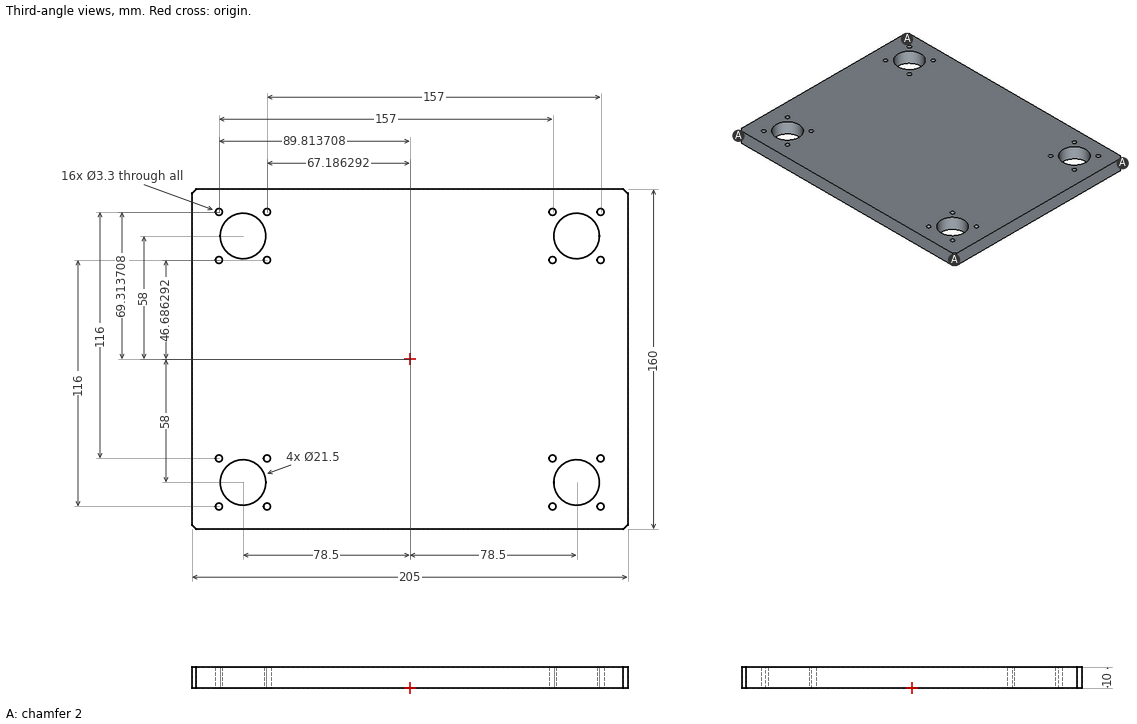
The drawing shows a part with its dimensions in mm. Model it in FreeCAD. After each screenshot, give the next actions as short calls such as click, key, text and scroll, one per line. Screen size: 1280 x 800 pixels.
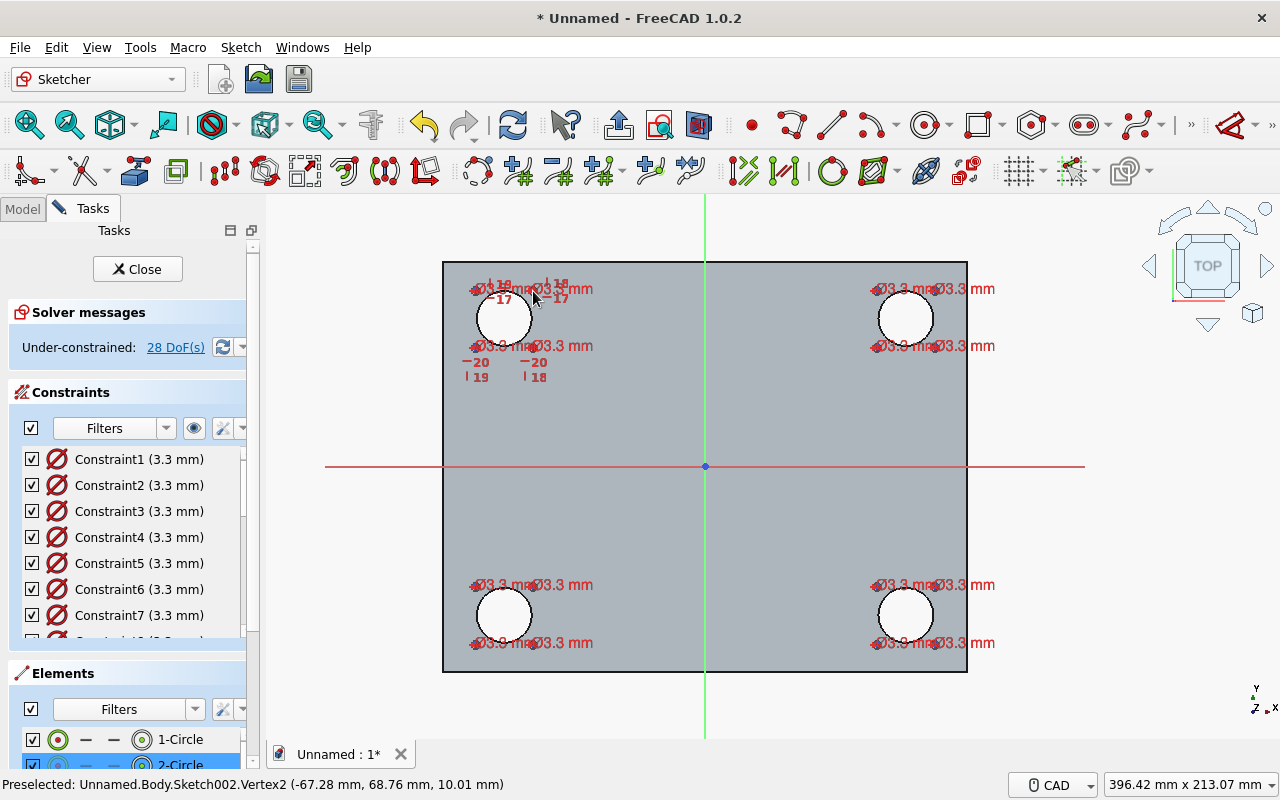
click(877, 291)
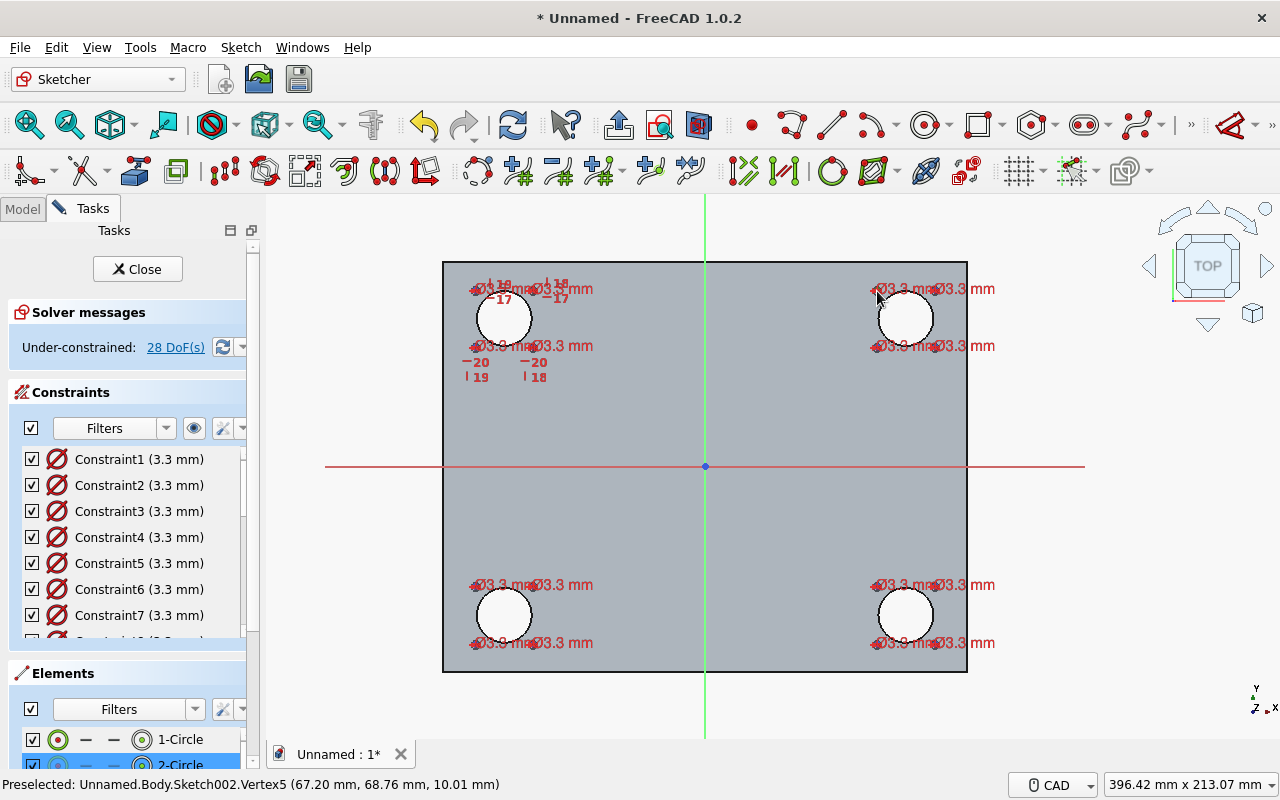
key(h)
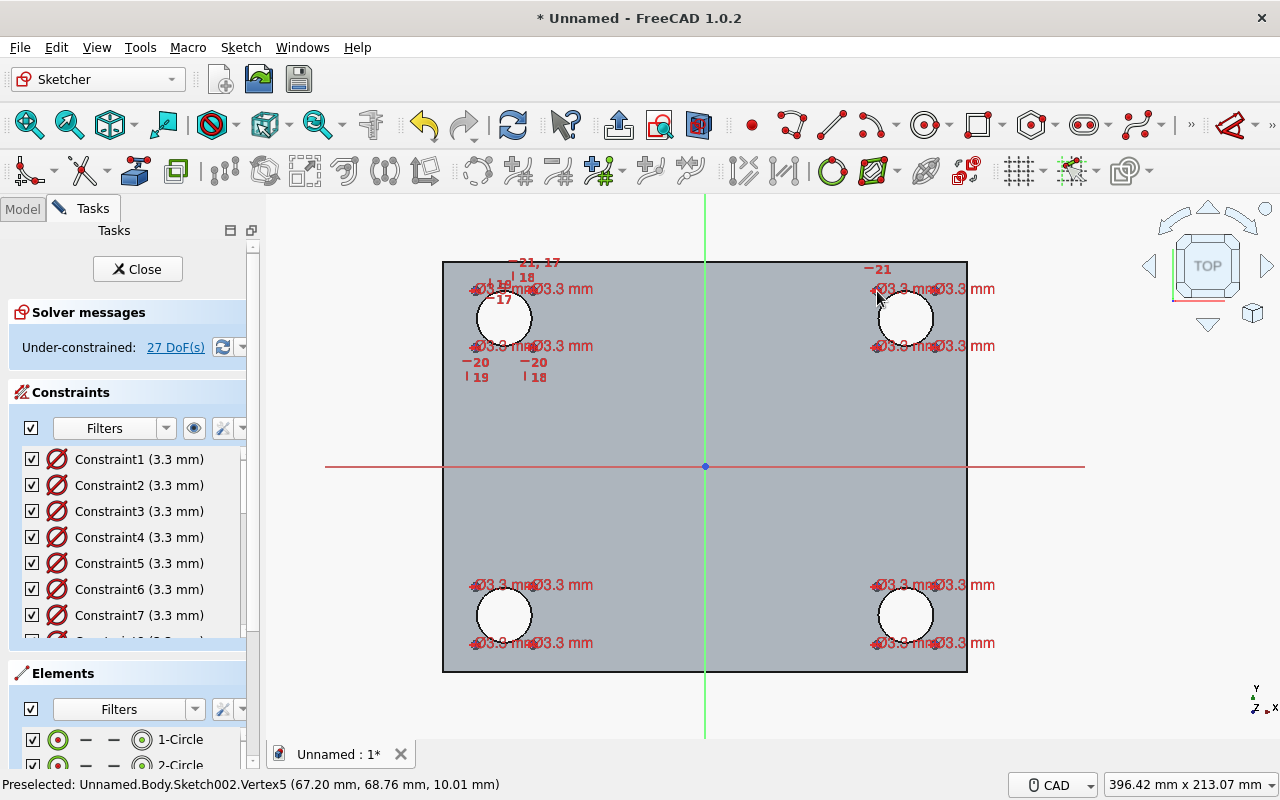
click(877, 291)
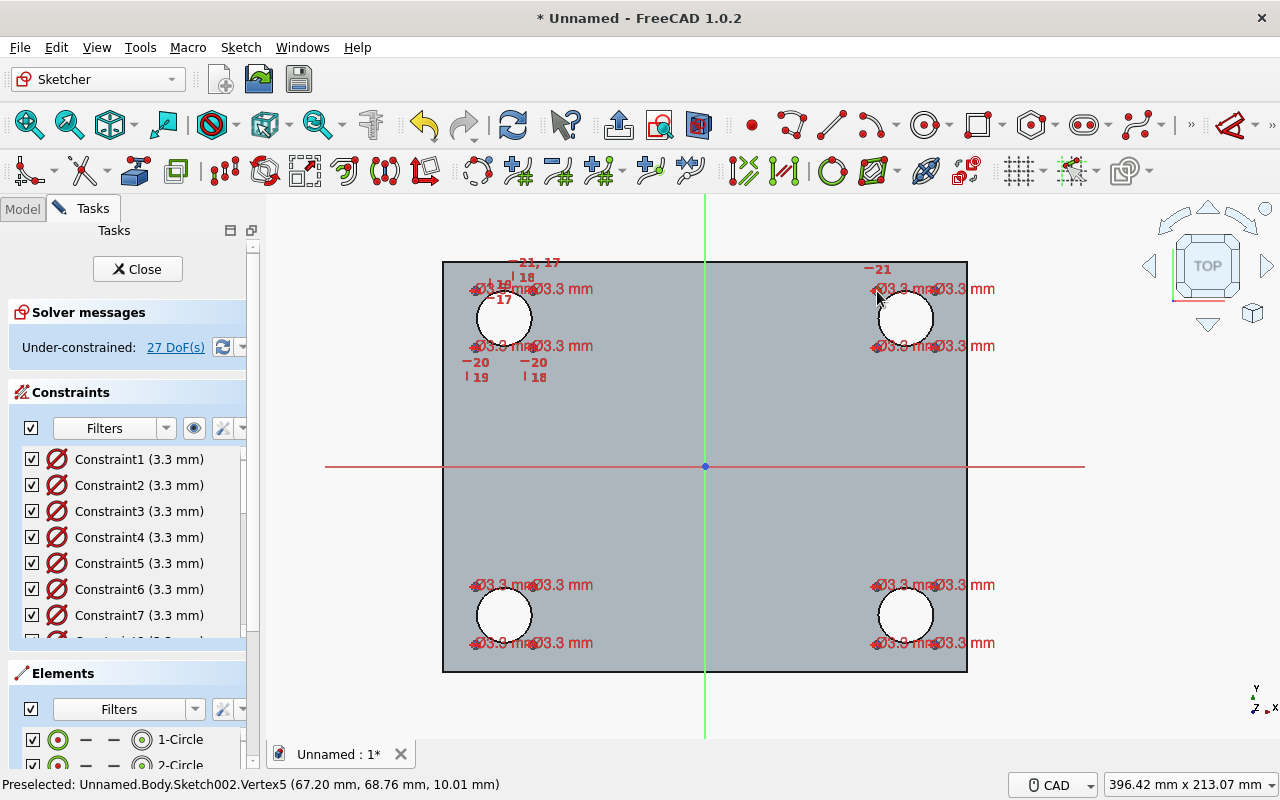
click(935, 291)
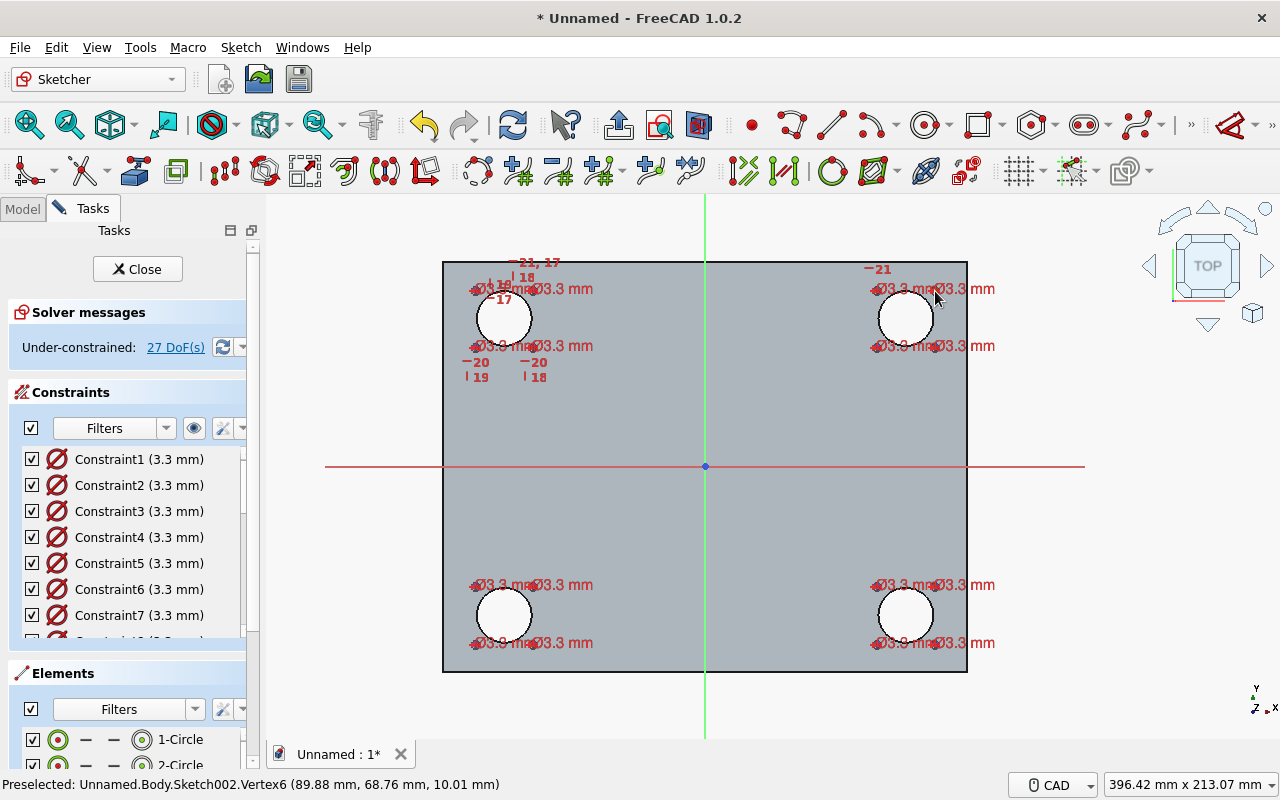
key(h)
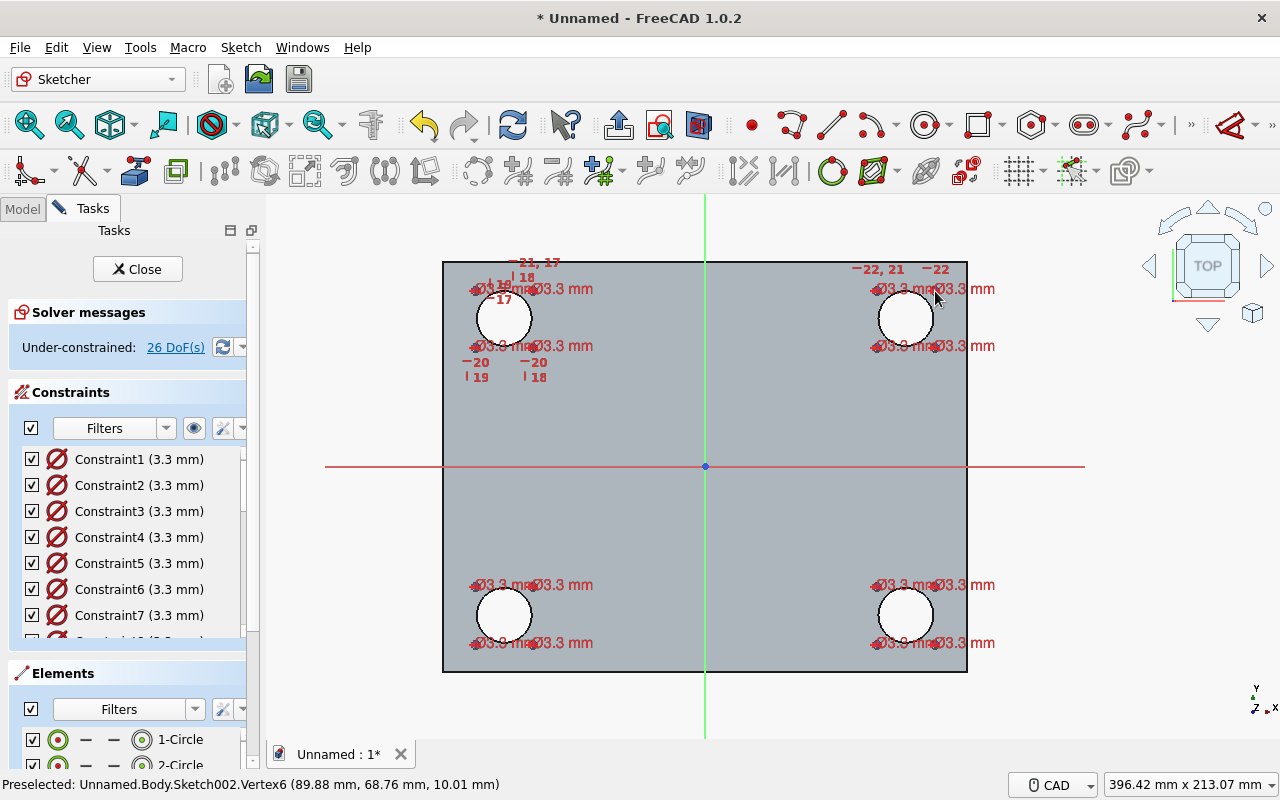
click(877, 291)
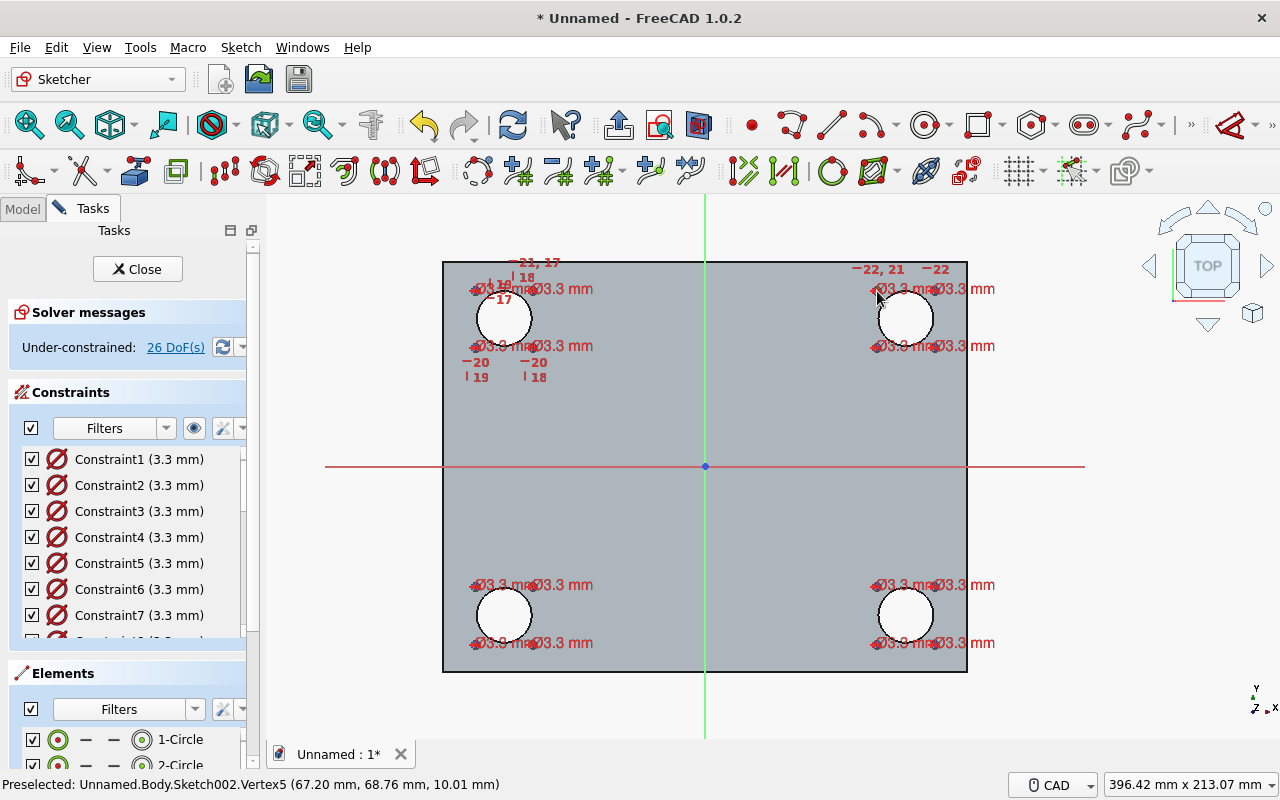
click(877, 348)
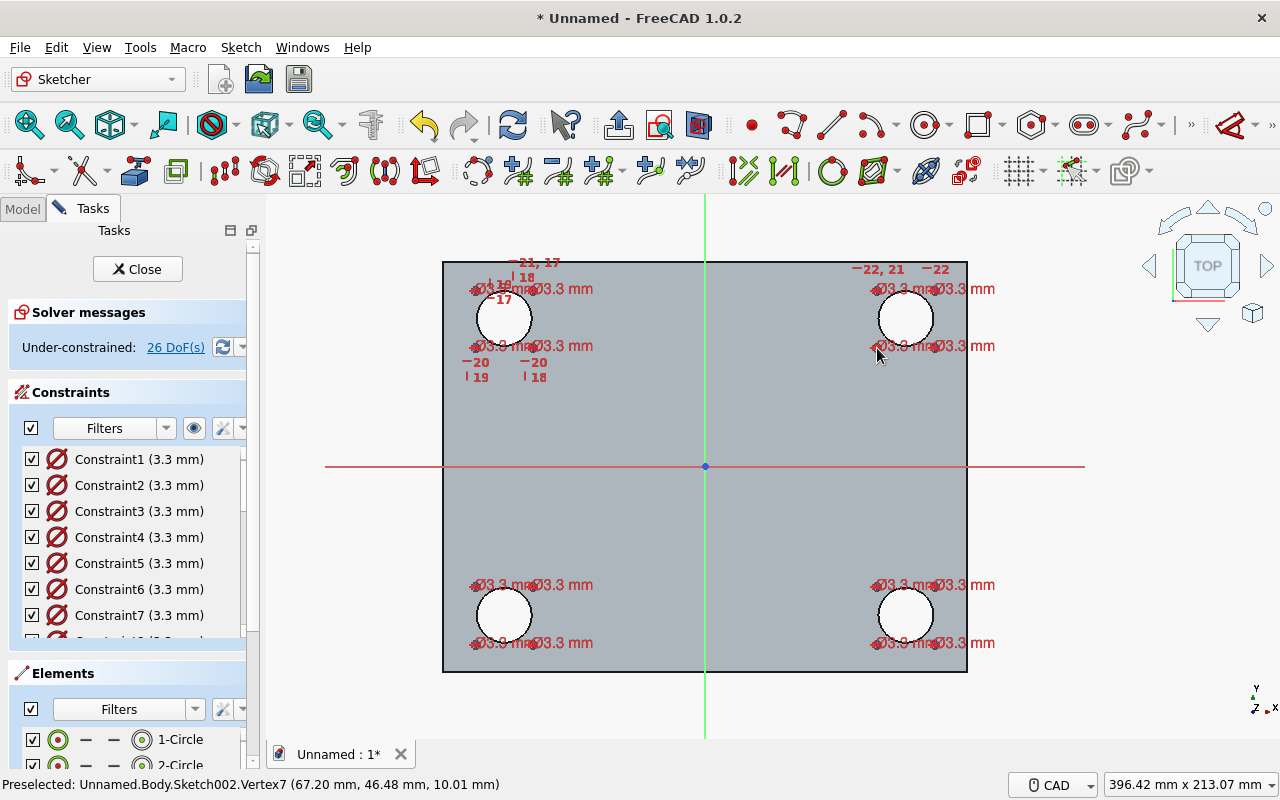
key(v)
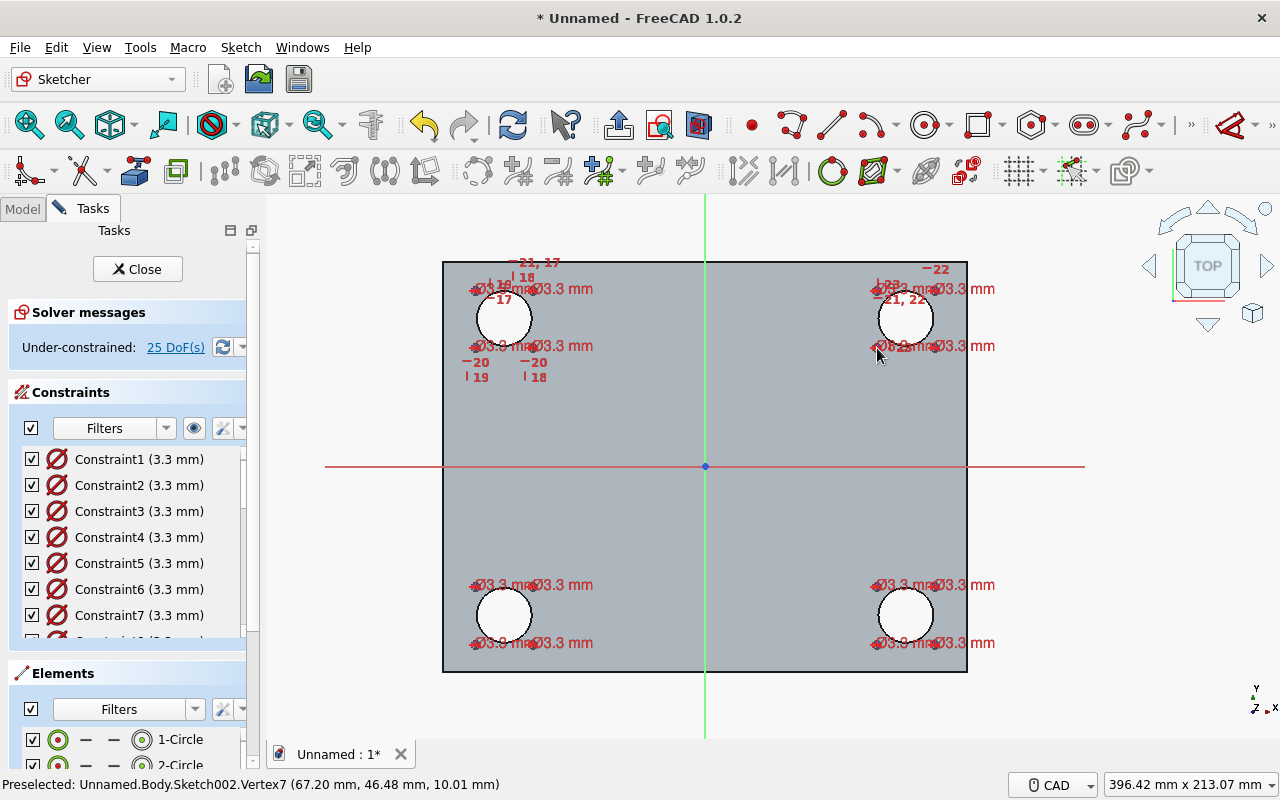
click(533, 348)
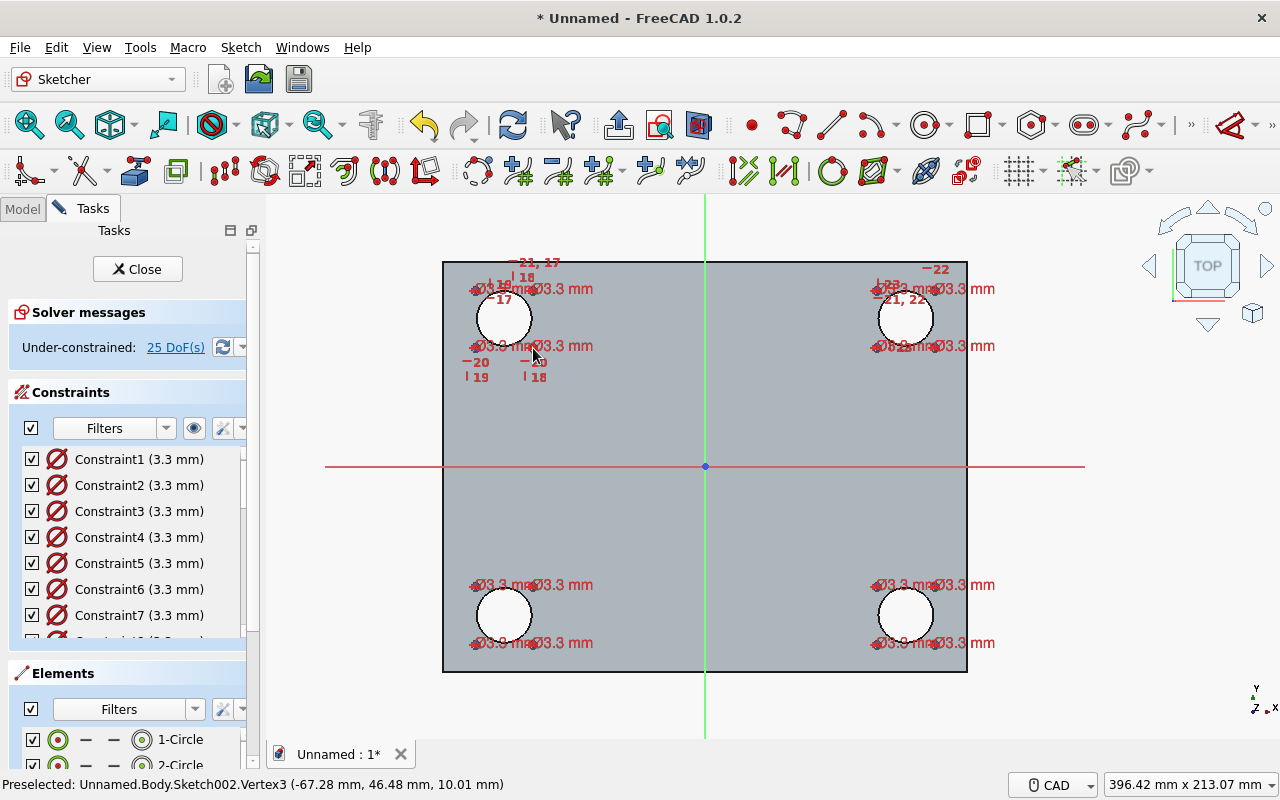
click(877, 348)